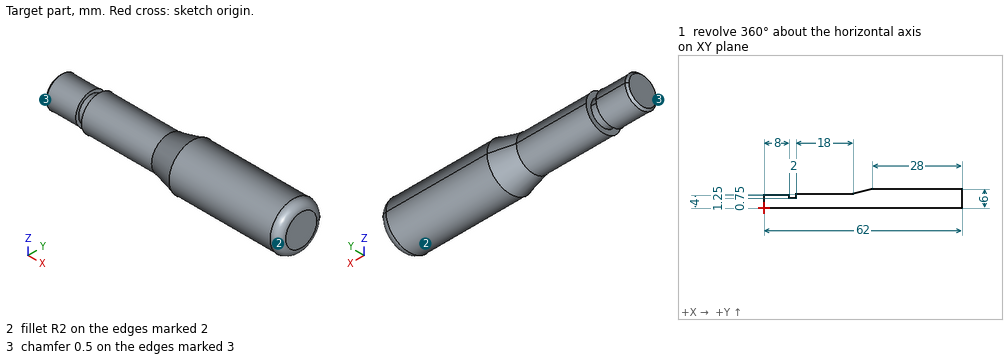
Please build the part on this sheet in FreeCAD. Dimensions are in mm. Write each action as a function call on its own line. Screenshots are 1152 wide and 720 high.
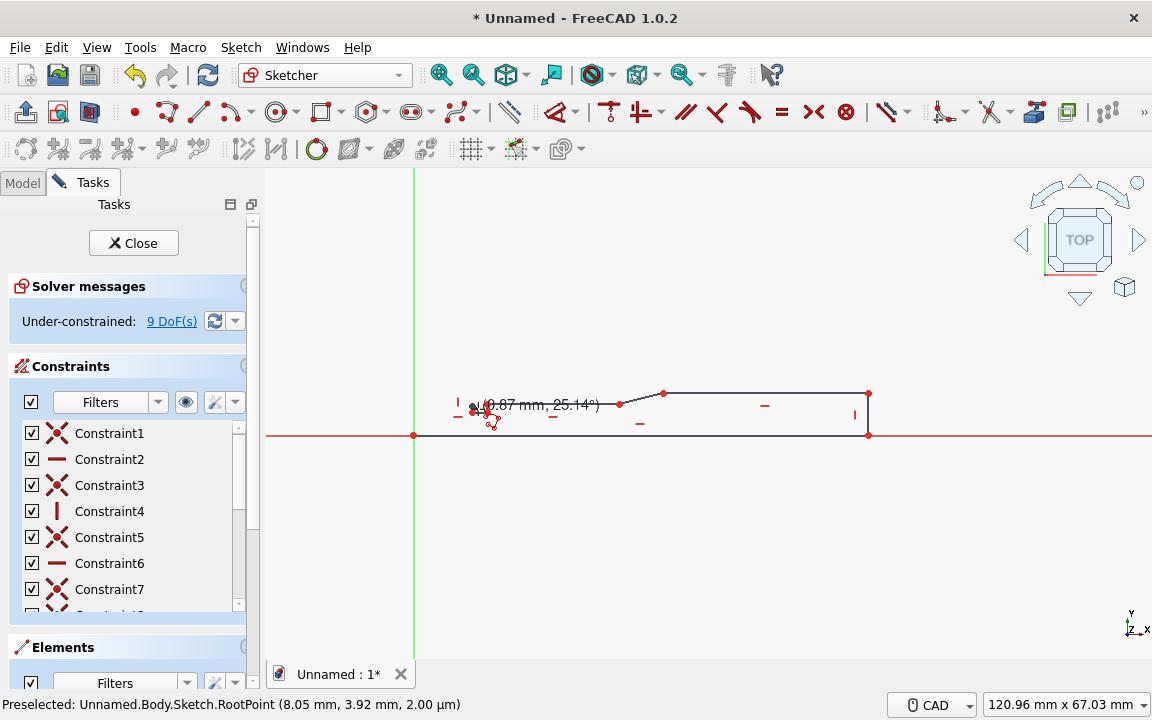
click(423, 407)
click(414, 436)
key(Escape)
key(Escape)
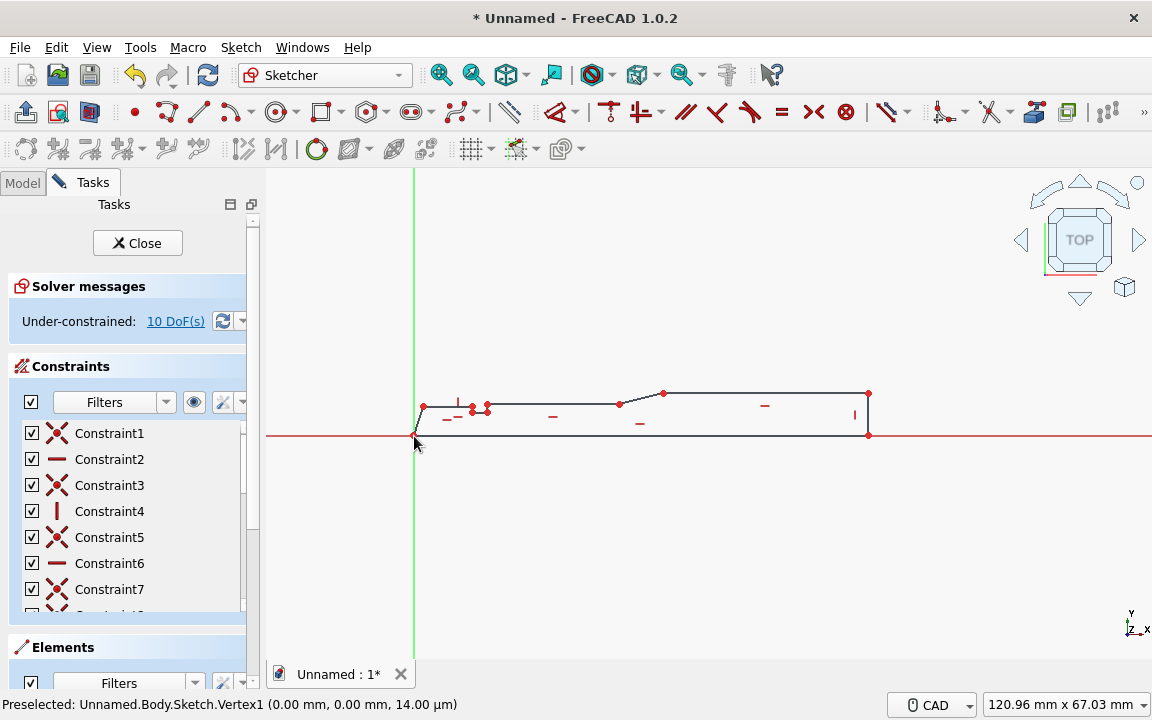
click(417, 424)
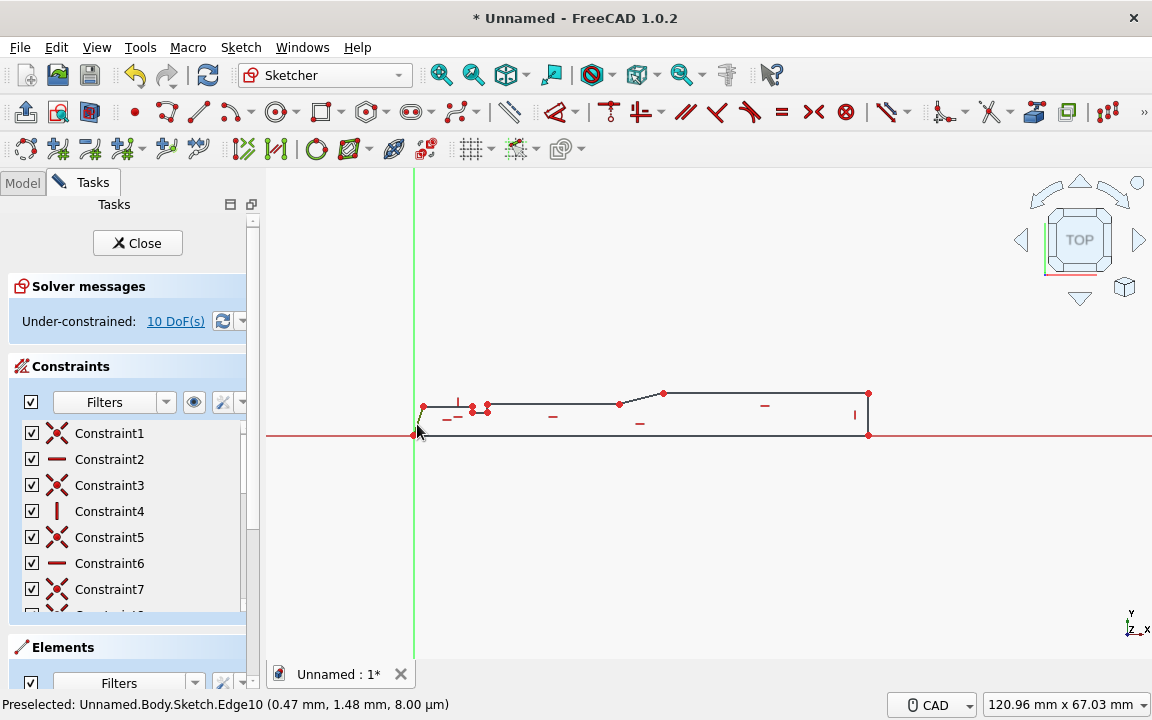
key(v)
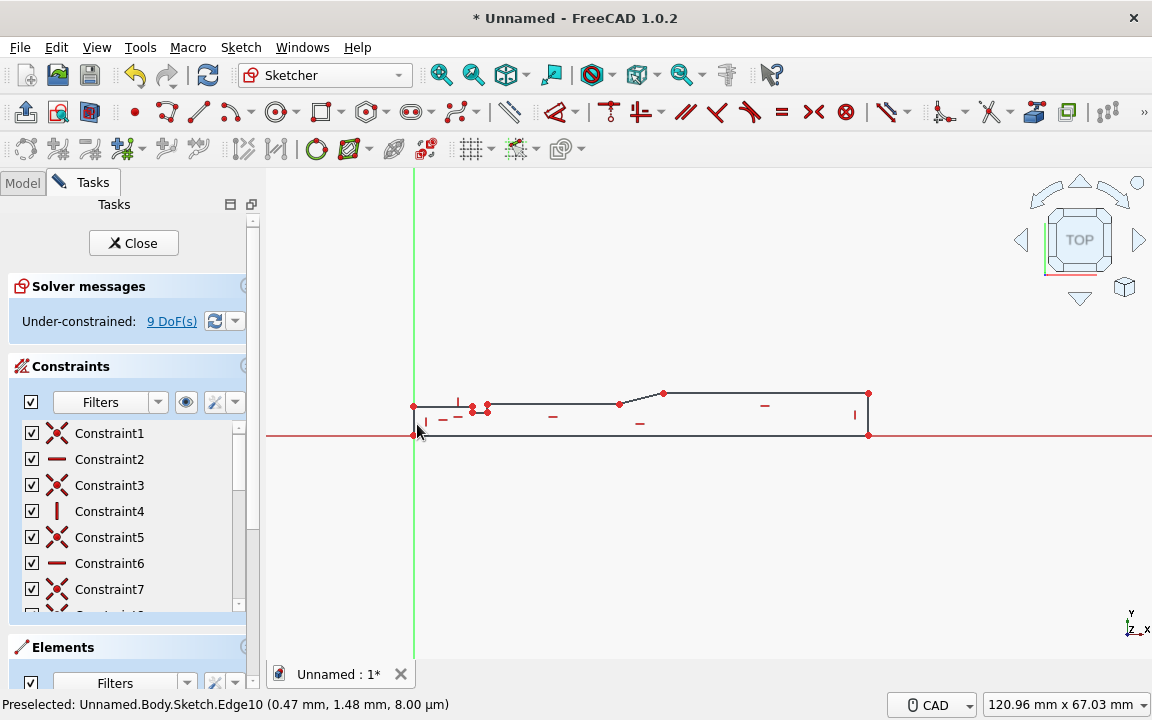
click(556, 112)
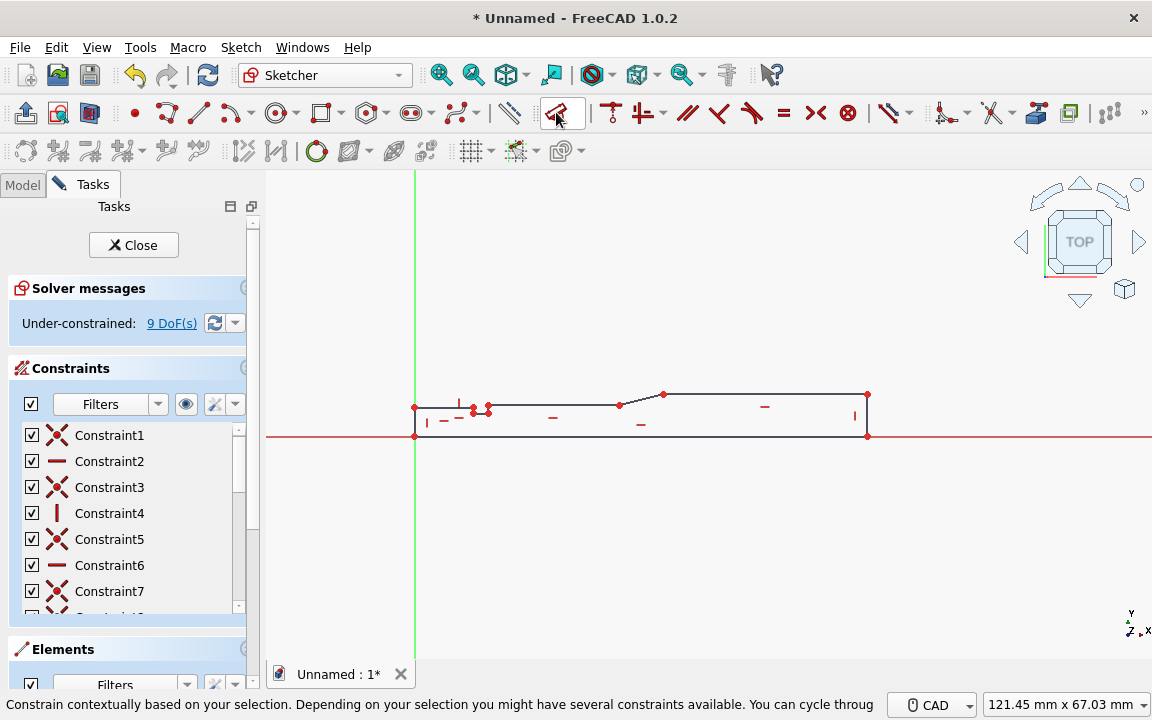
click(867, 424)
click(901, 416)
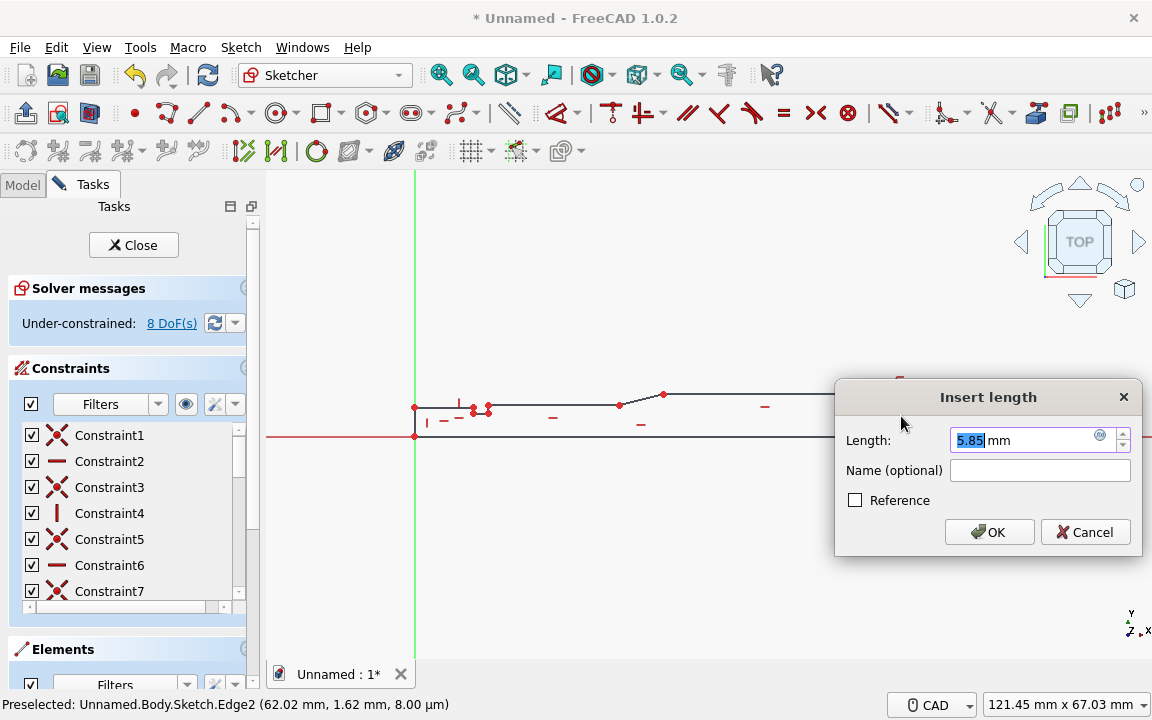
text(6)
key(Return)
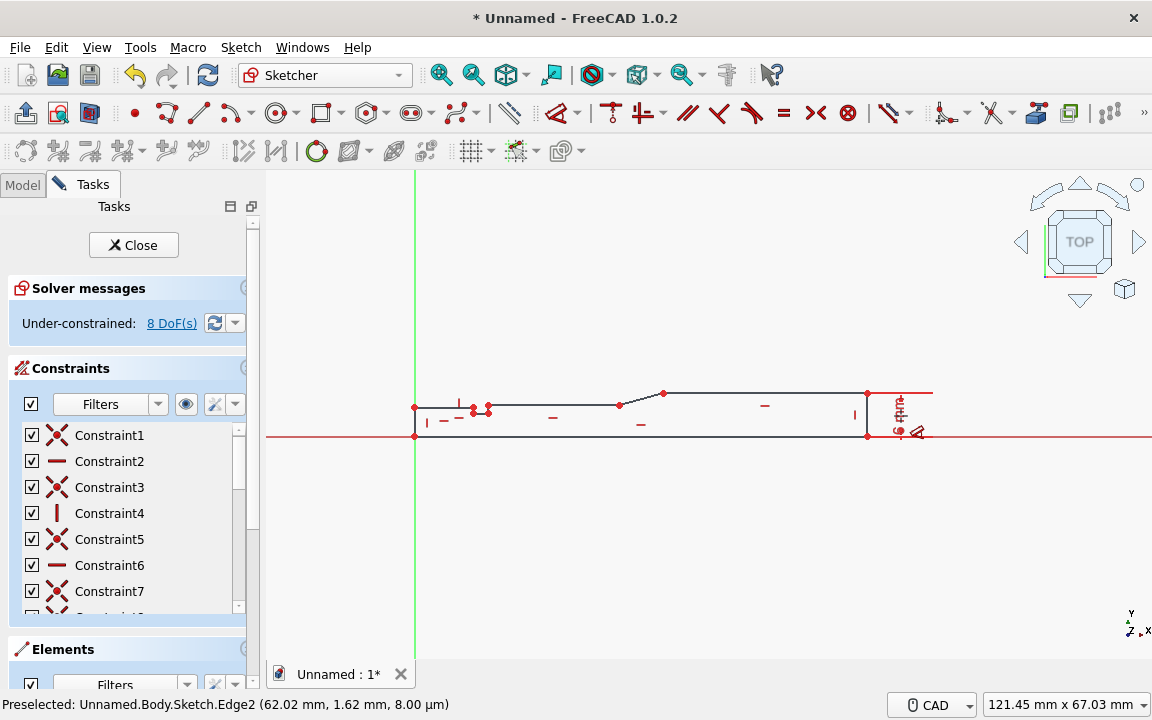
scroll(481, 414, up, 6)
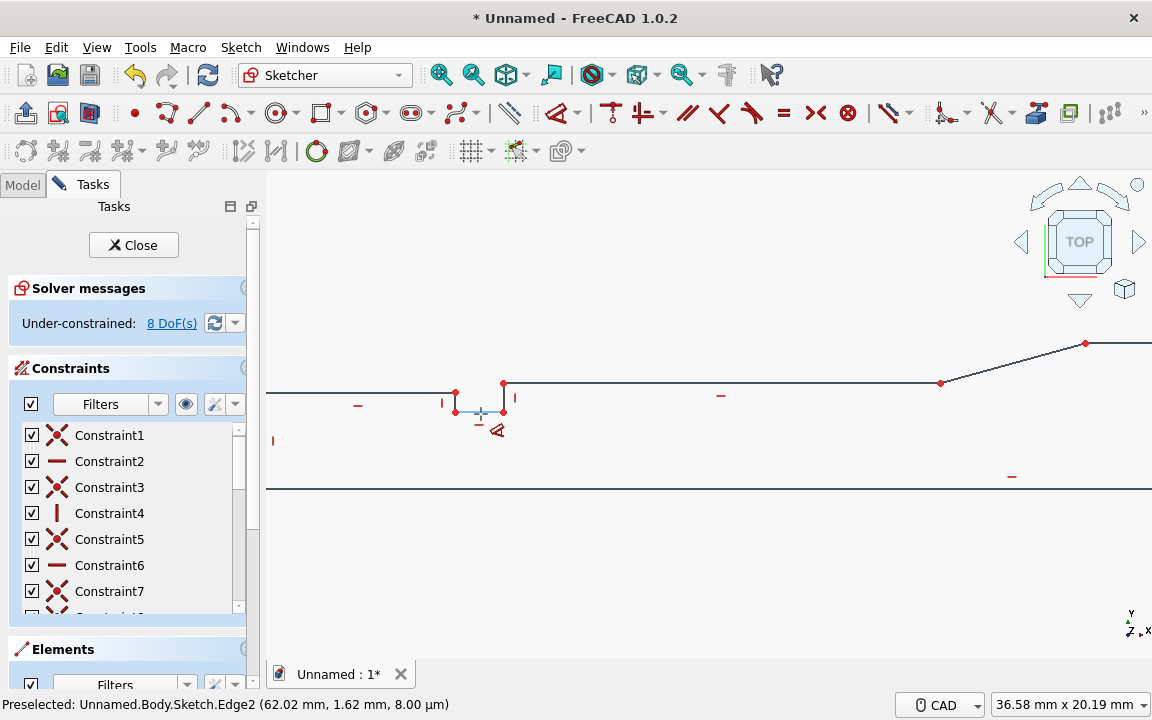
click(479, 412)
click(479, 378)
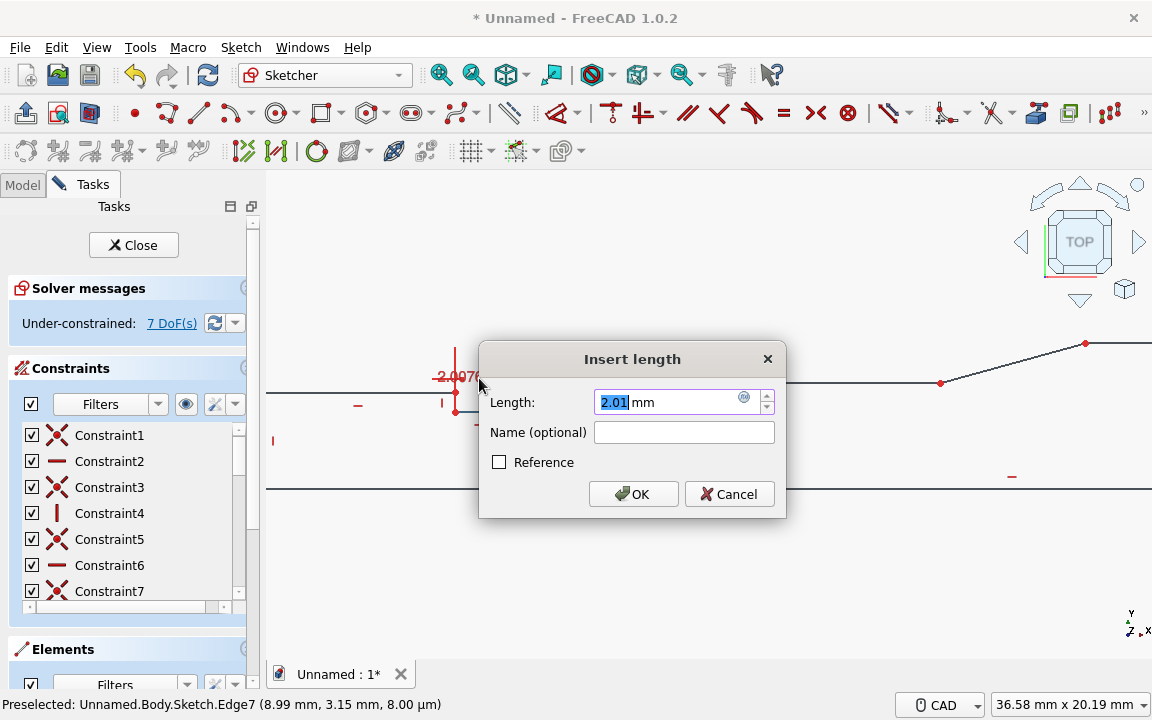
text(2)
key(Return)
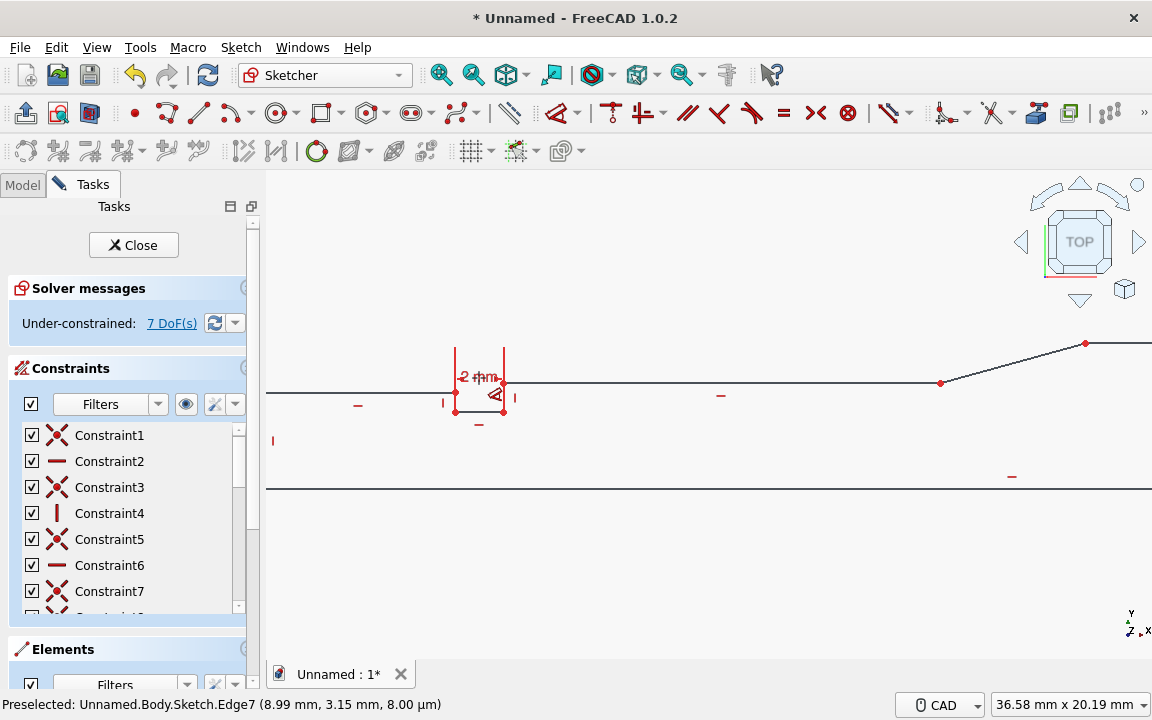
click(397, 393)
click(375, 359)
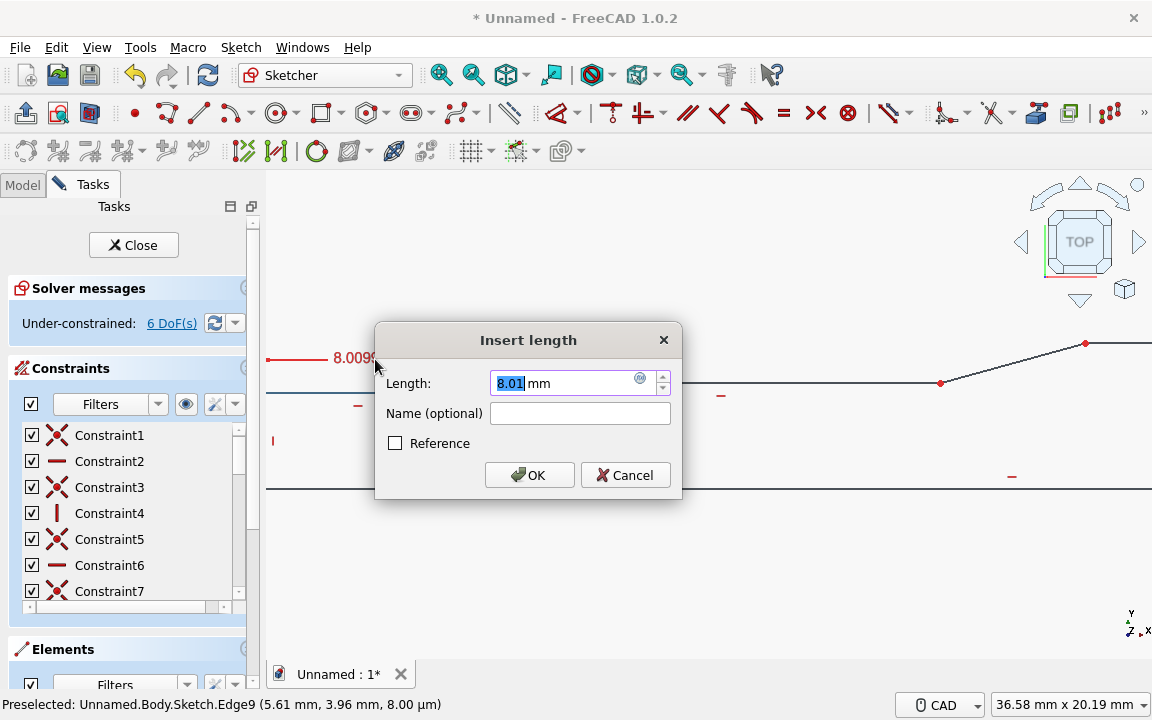
text(8)
key(Return)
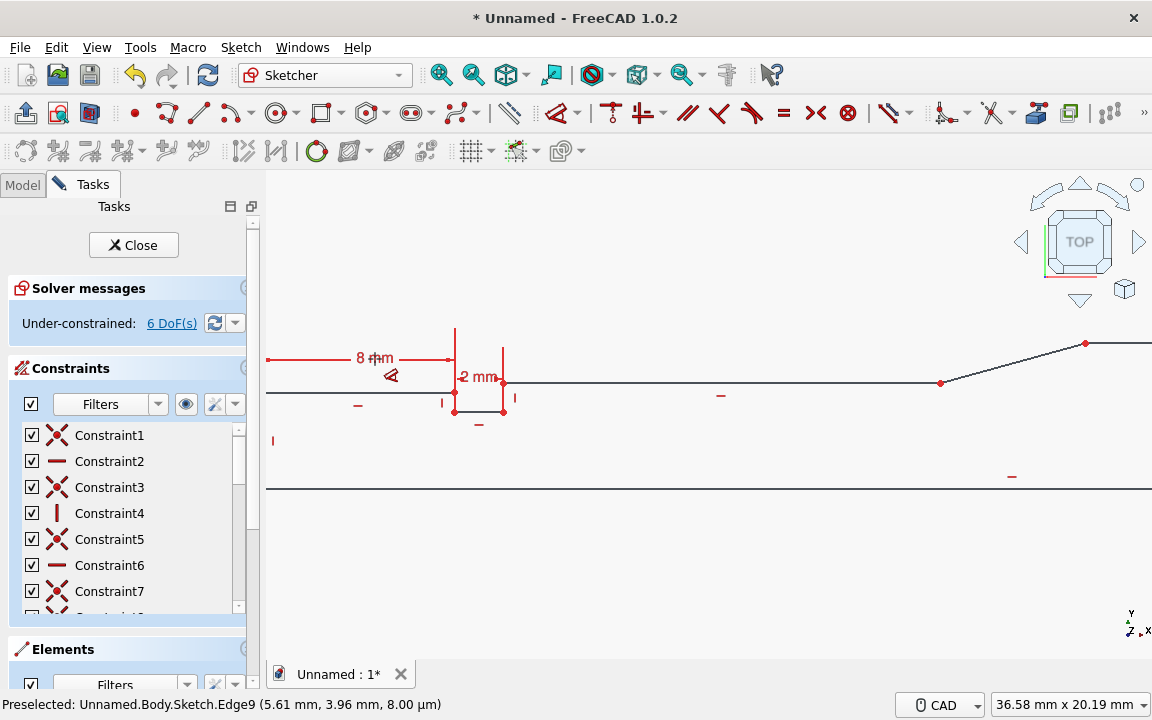
scroll(480, 414, down, 6)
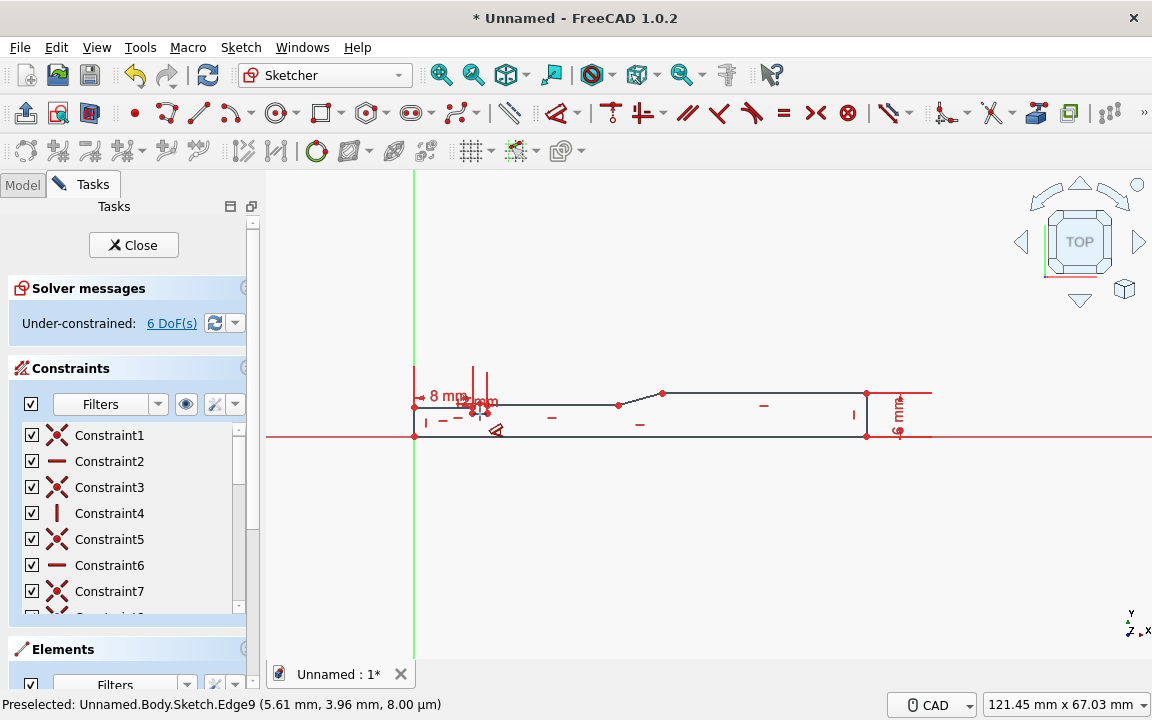
scroll(414, 417, up, 3)